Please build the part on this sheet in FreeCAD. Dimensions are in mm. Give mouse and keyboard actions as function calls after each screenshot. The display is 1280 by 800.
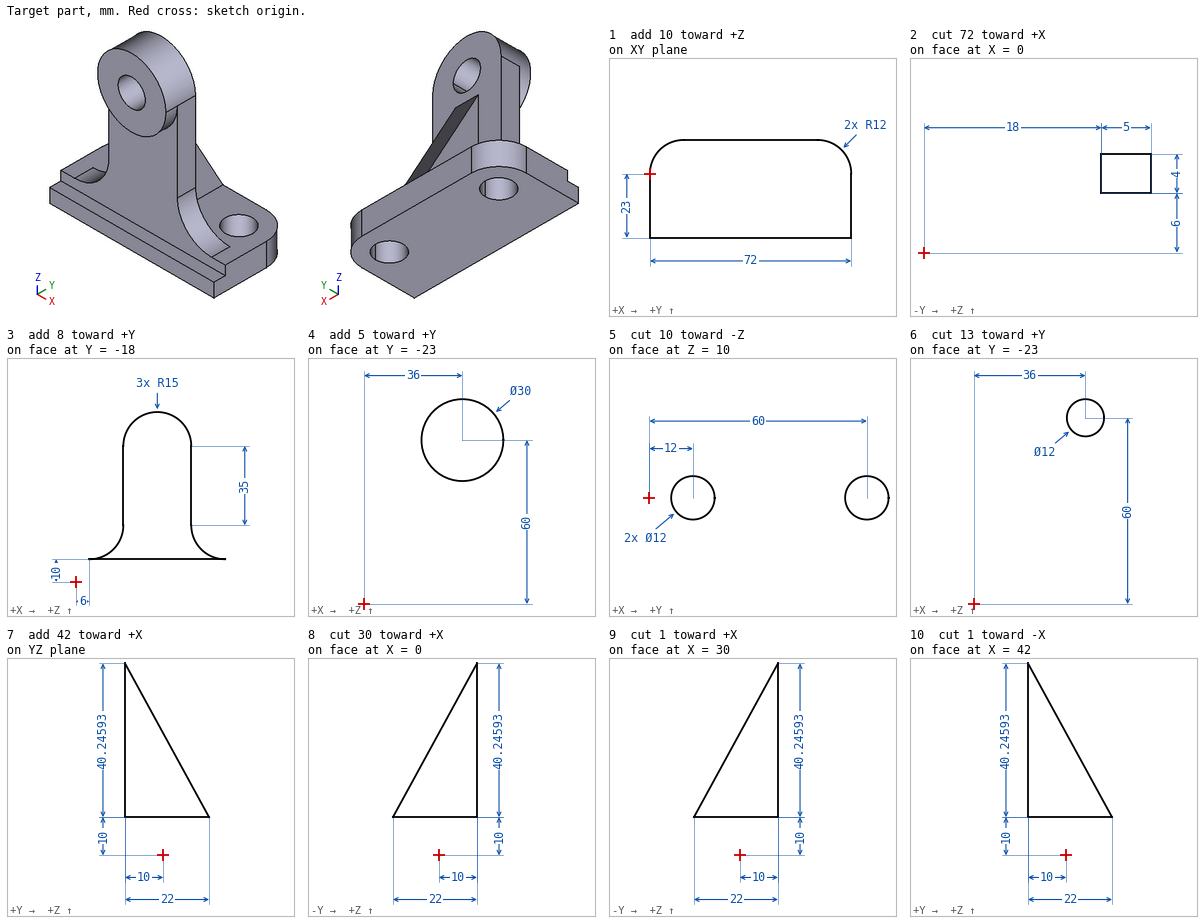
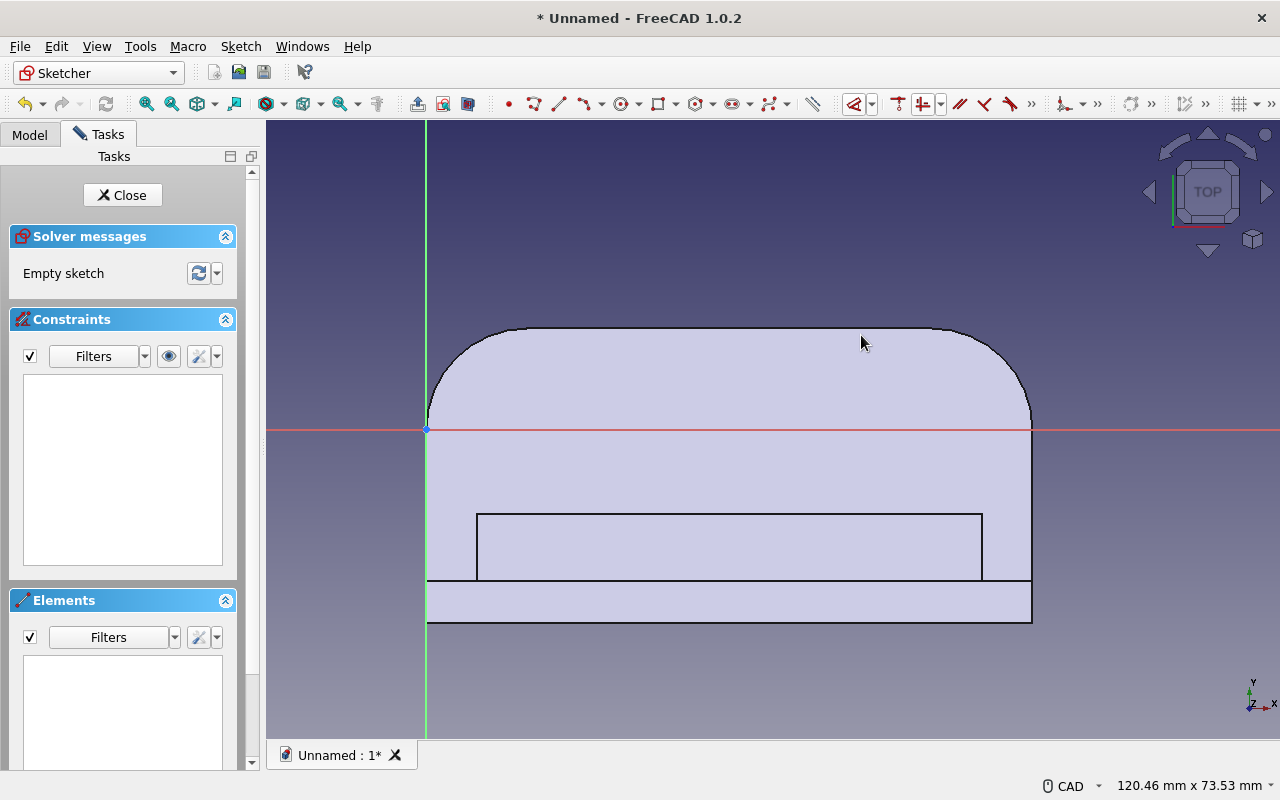
click(620, 104)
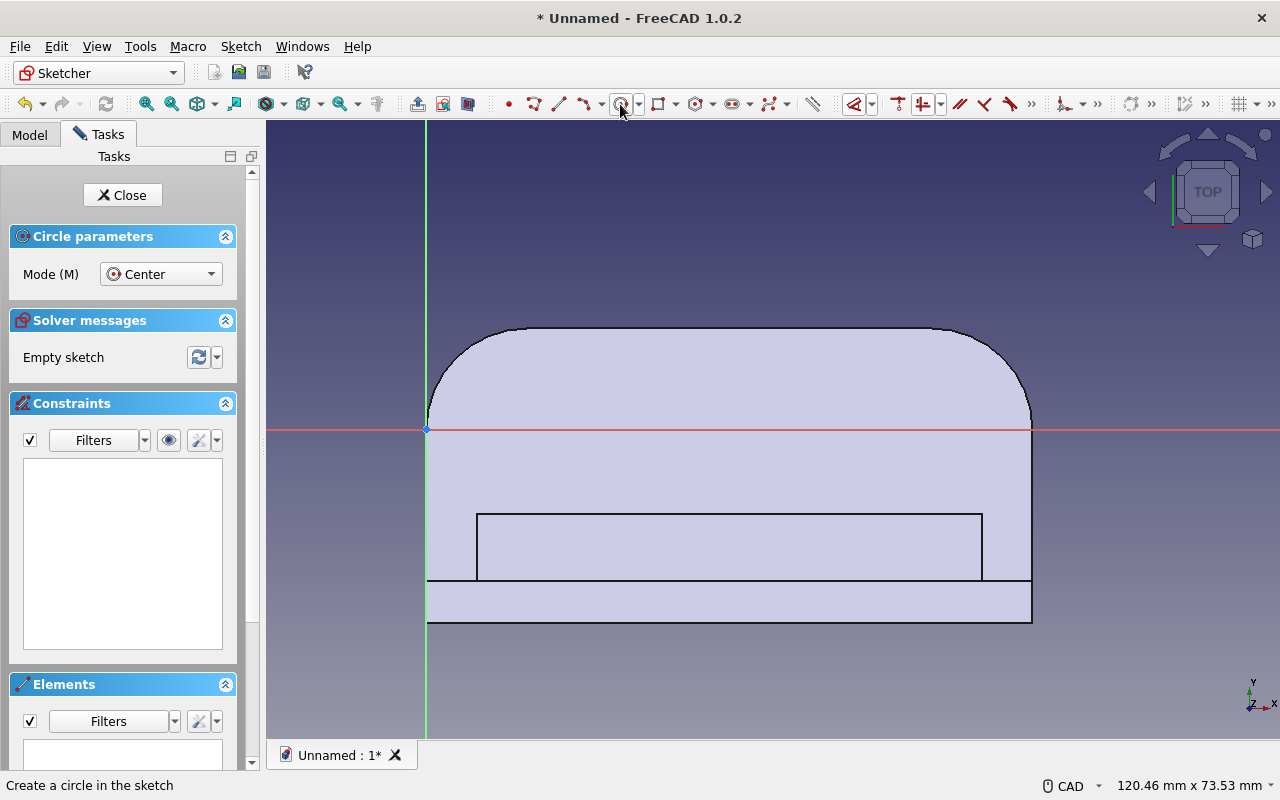
click(527, 430)
move(563, 394)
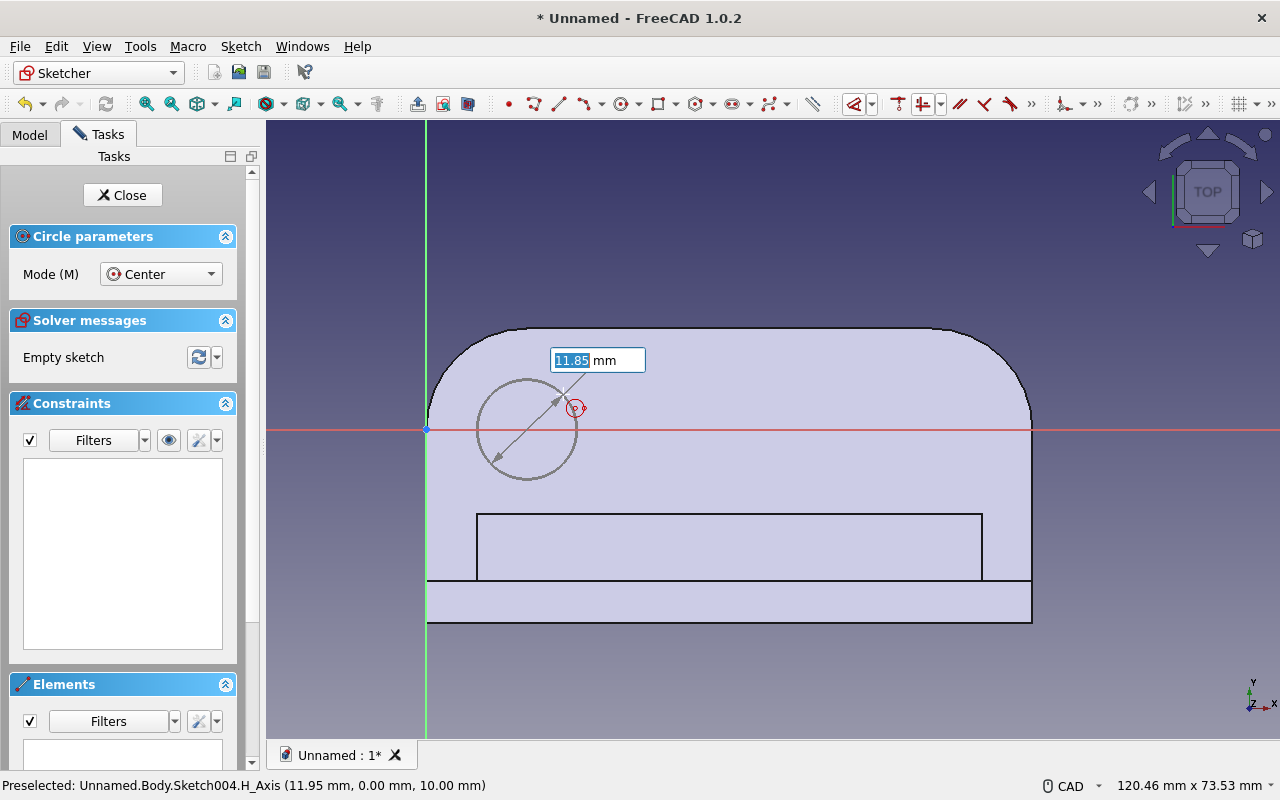
text(12)
key(Return)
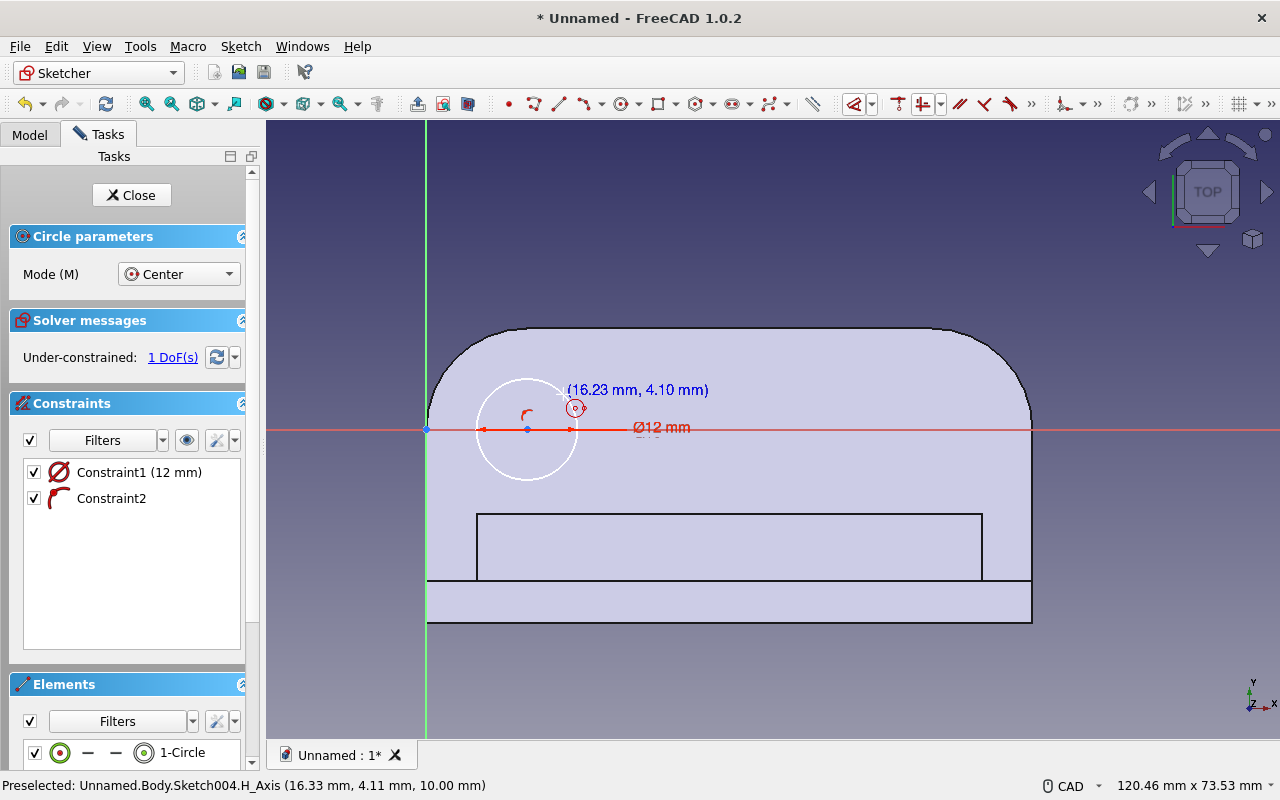
click(931, 430)
move(967, 394)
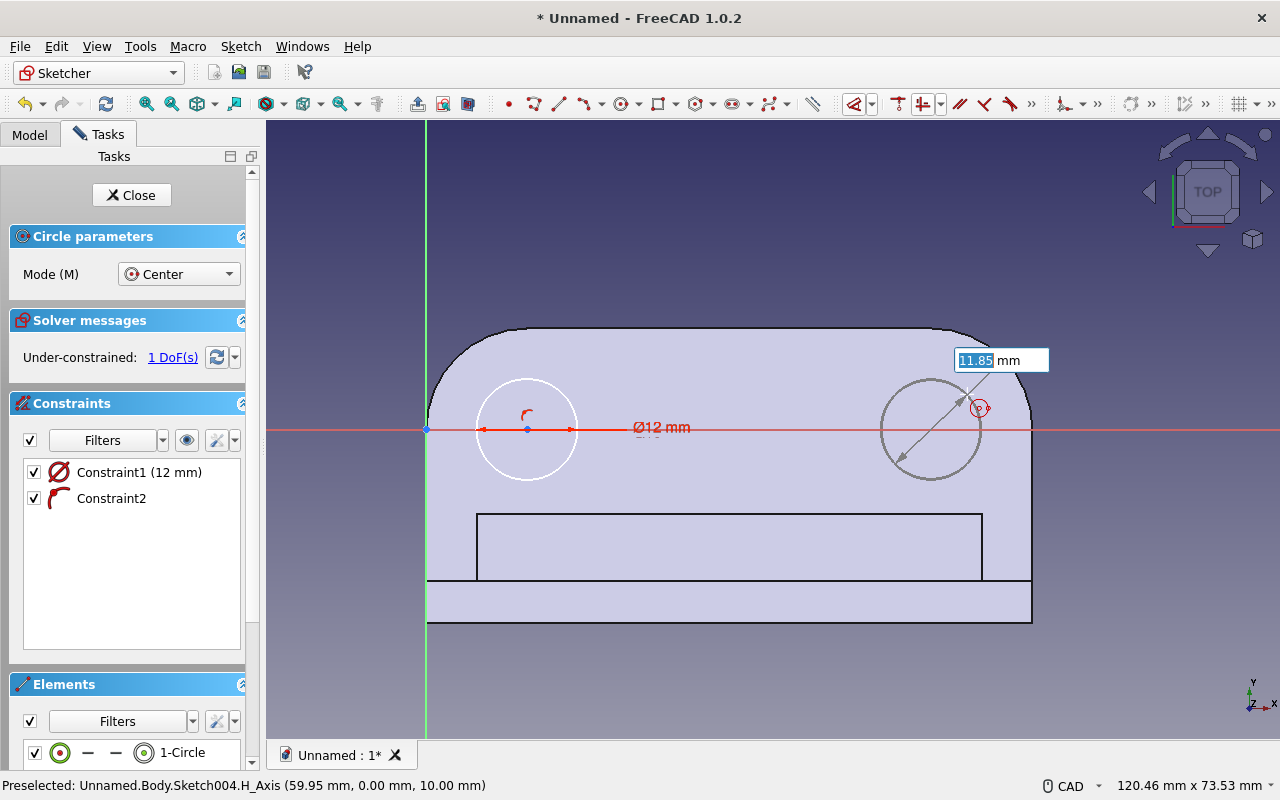
text(12)
key(Return)
key(Escape)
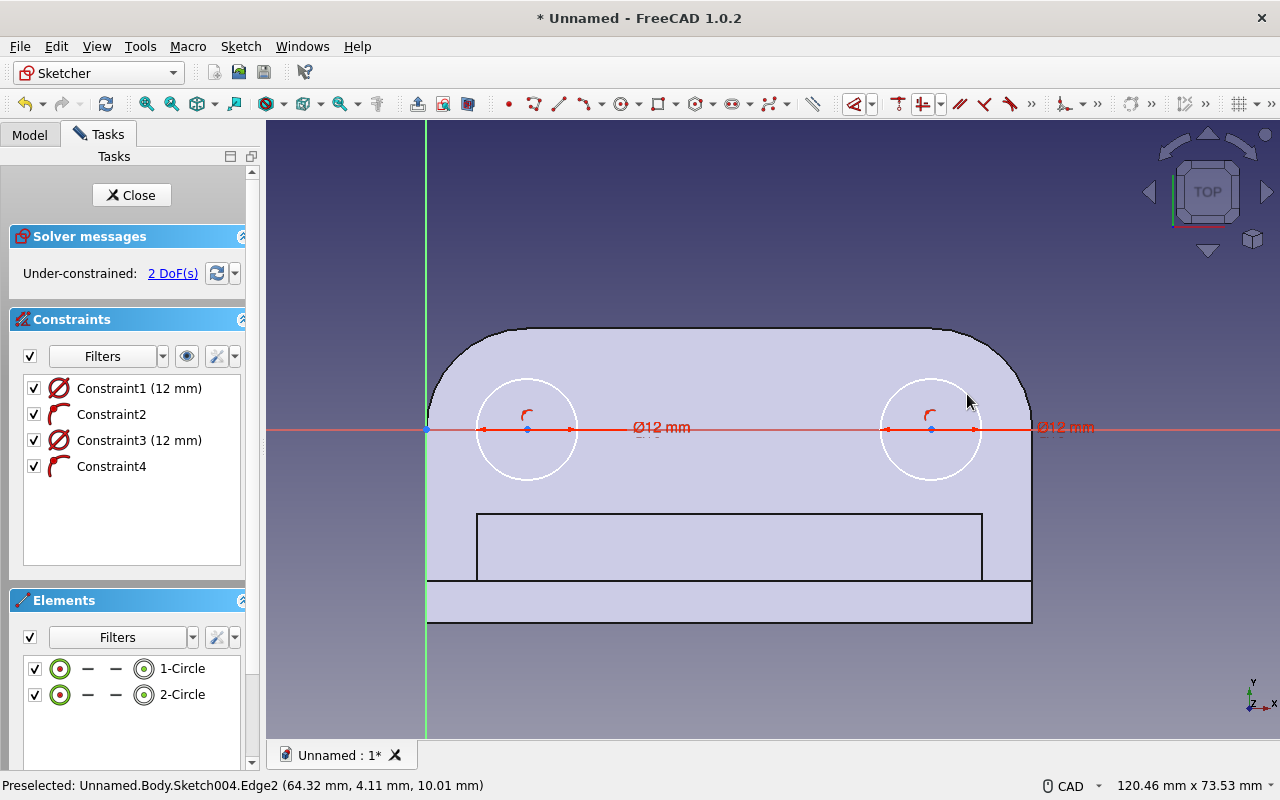
click(527, 430)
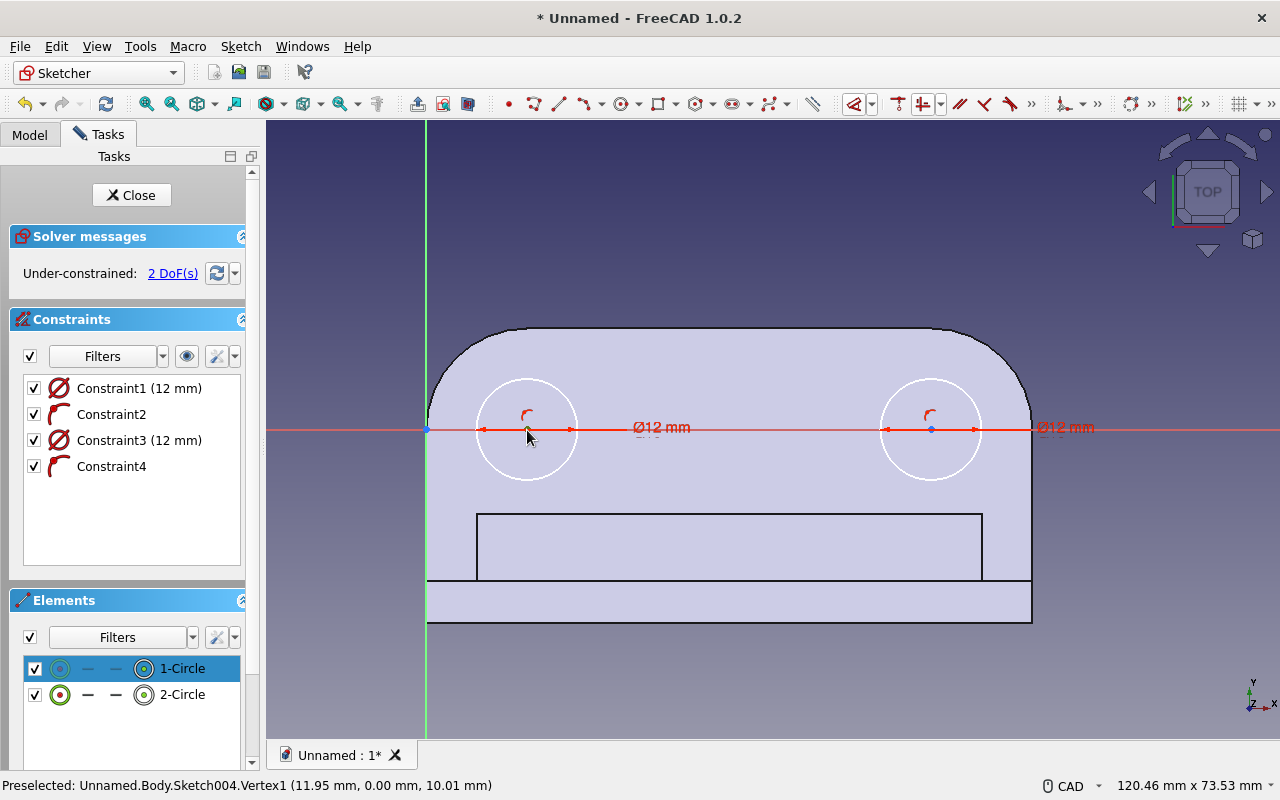
key(l)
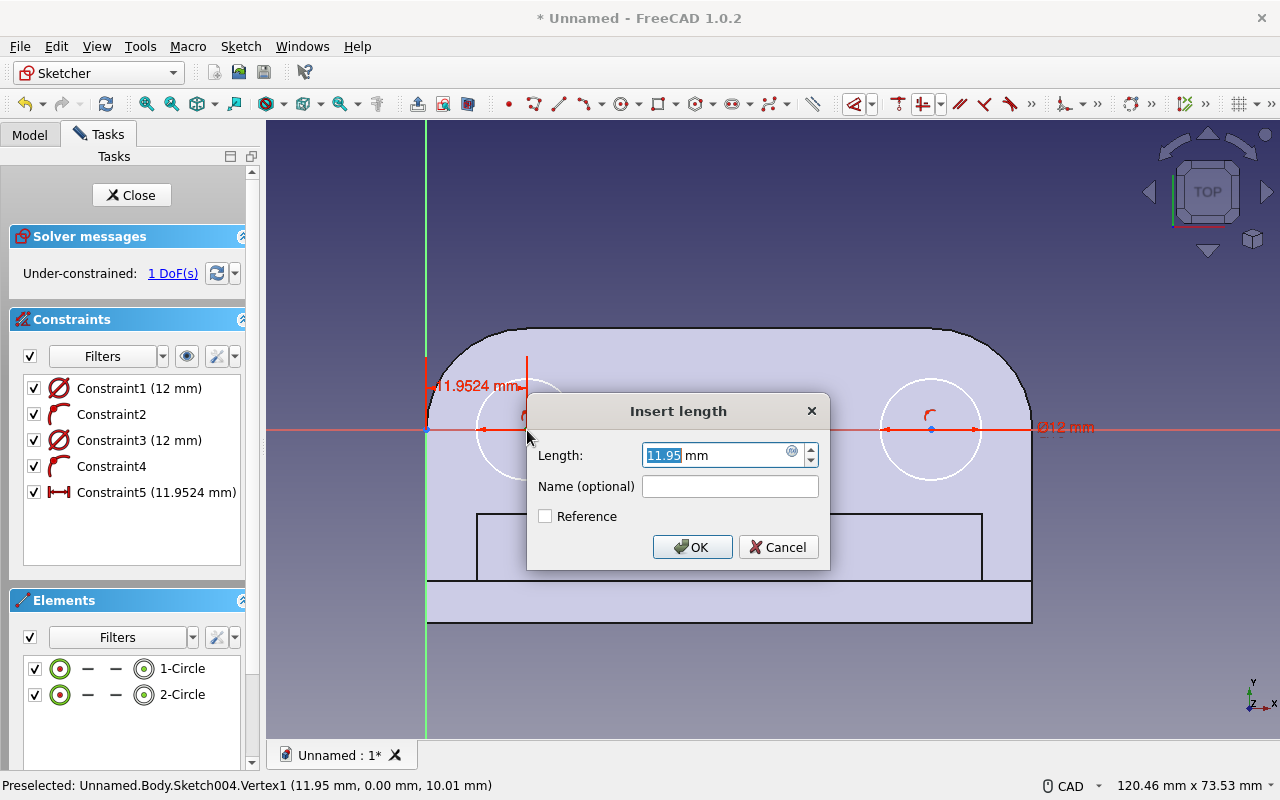
text(12)
key(Return)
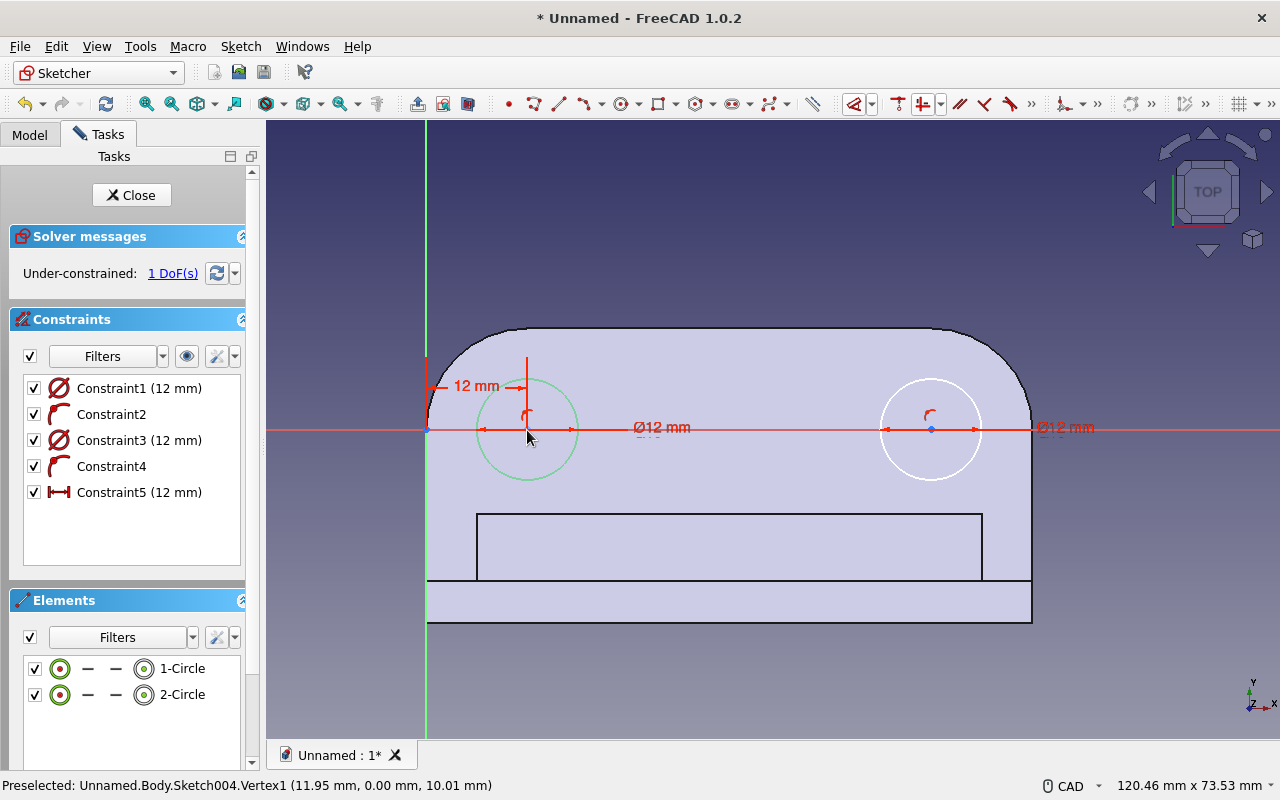
click(931, 430)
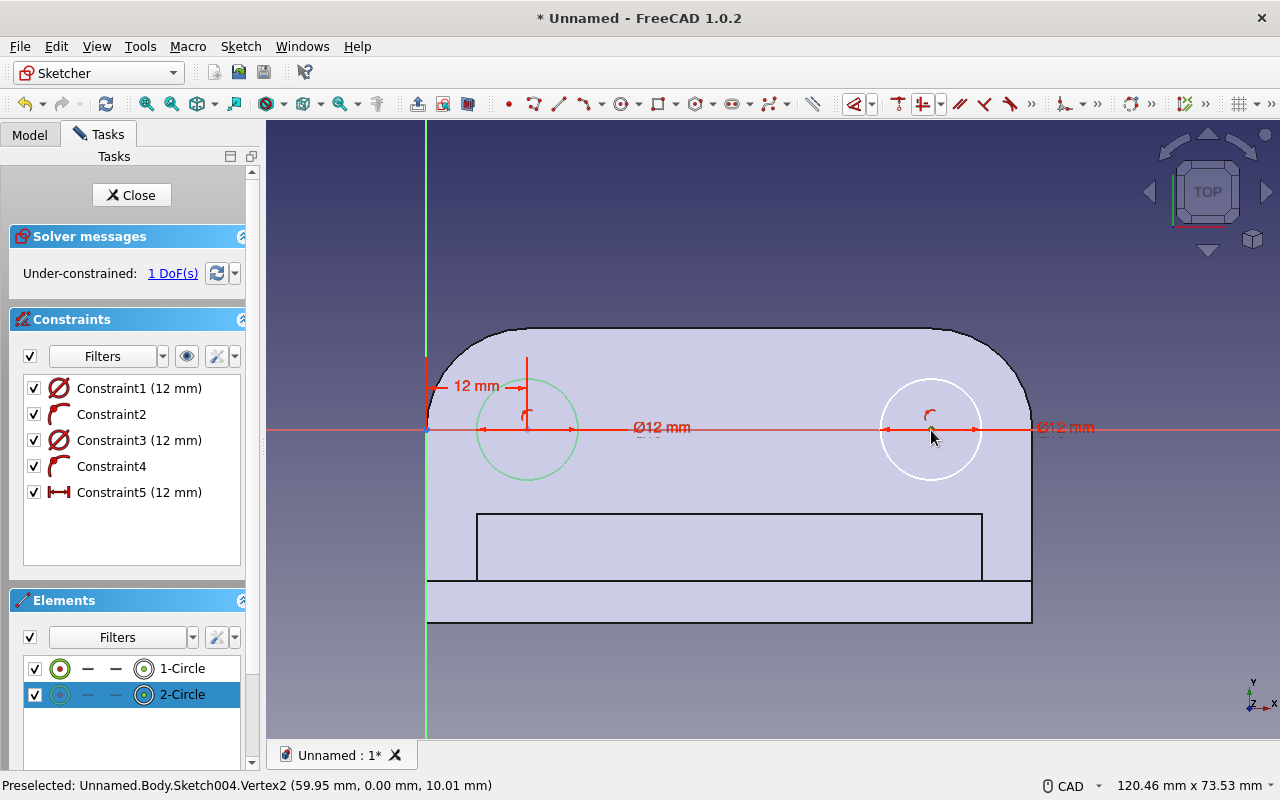
key(l)